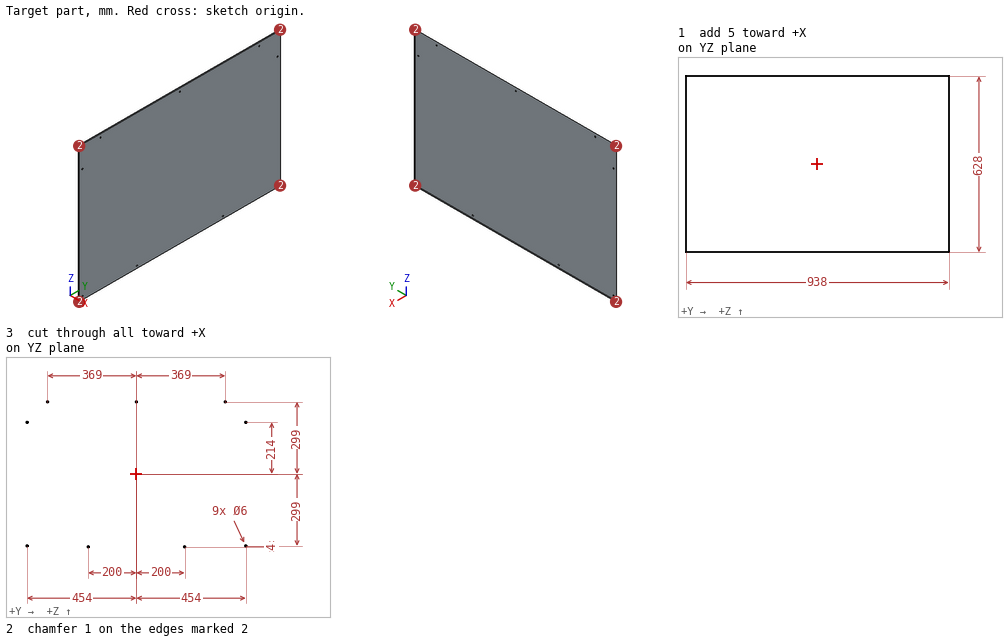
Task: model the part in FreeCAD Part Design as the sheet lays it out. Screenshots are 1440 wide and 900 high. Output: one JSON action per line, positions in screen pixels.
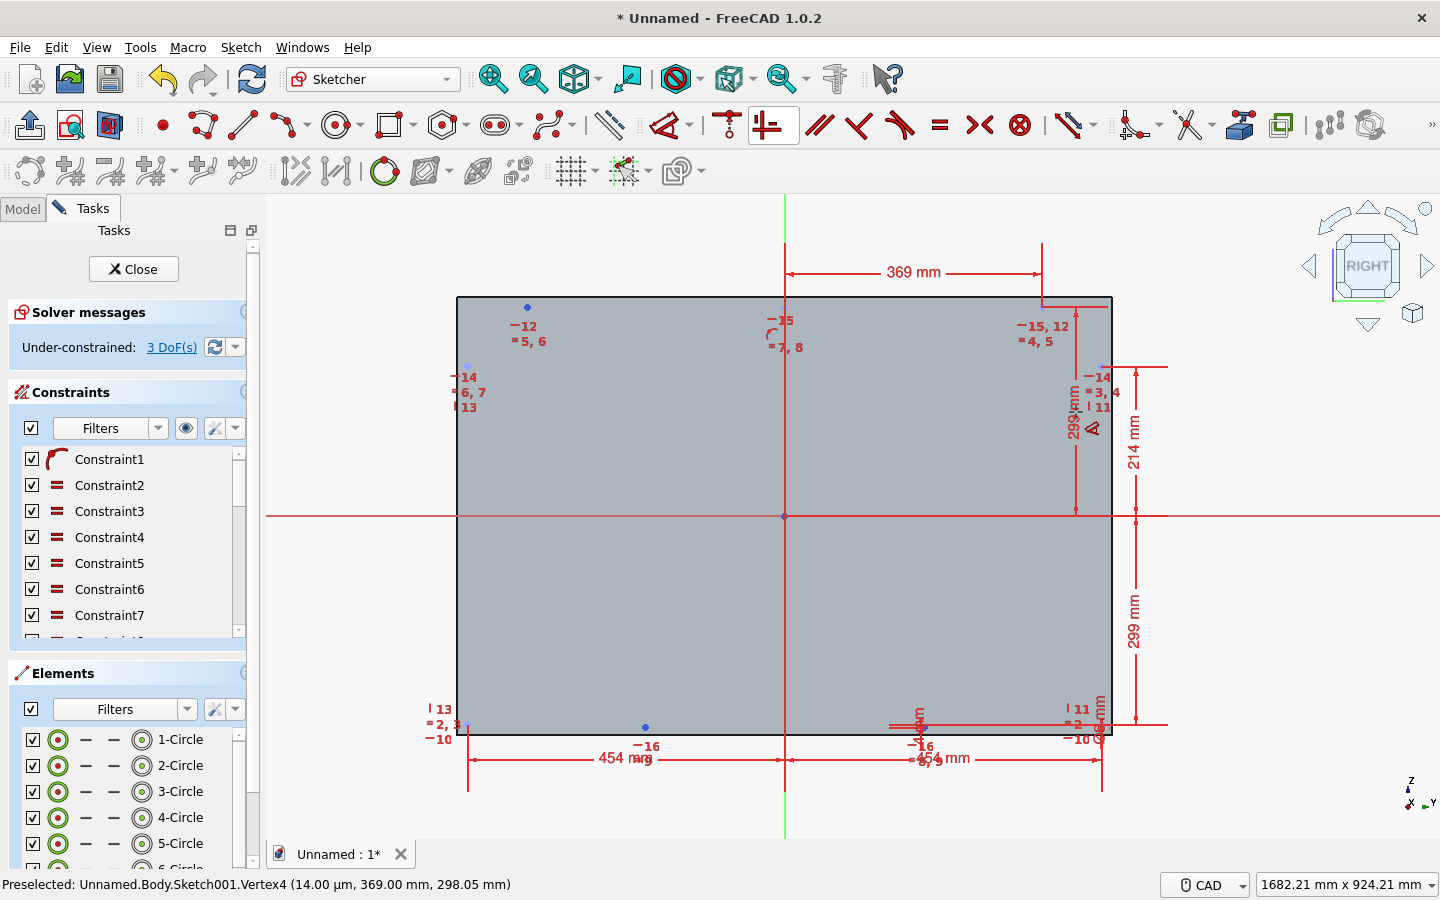
{"action": "left_click", "coordinate": [527, 307]}
{"action": "left_click", "coordinate": [656, 273]}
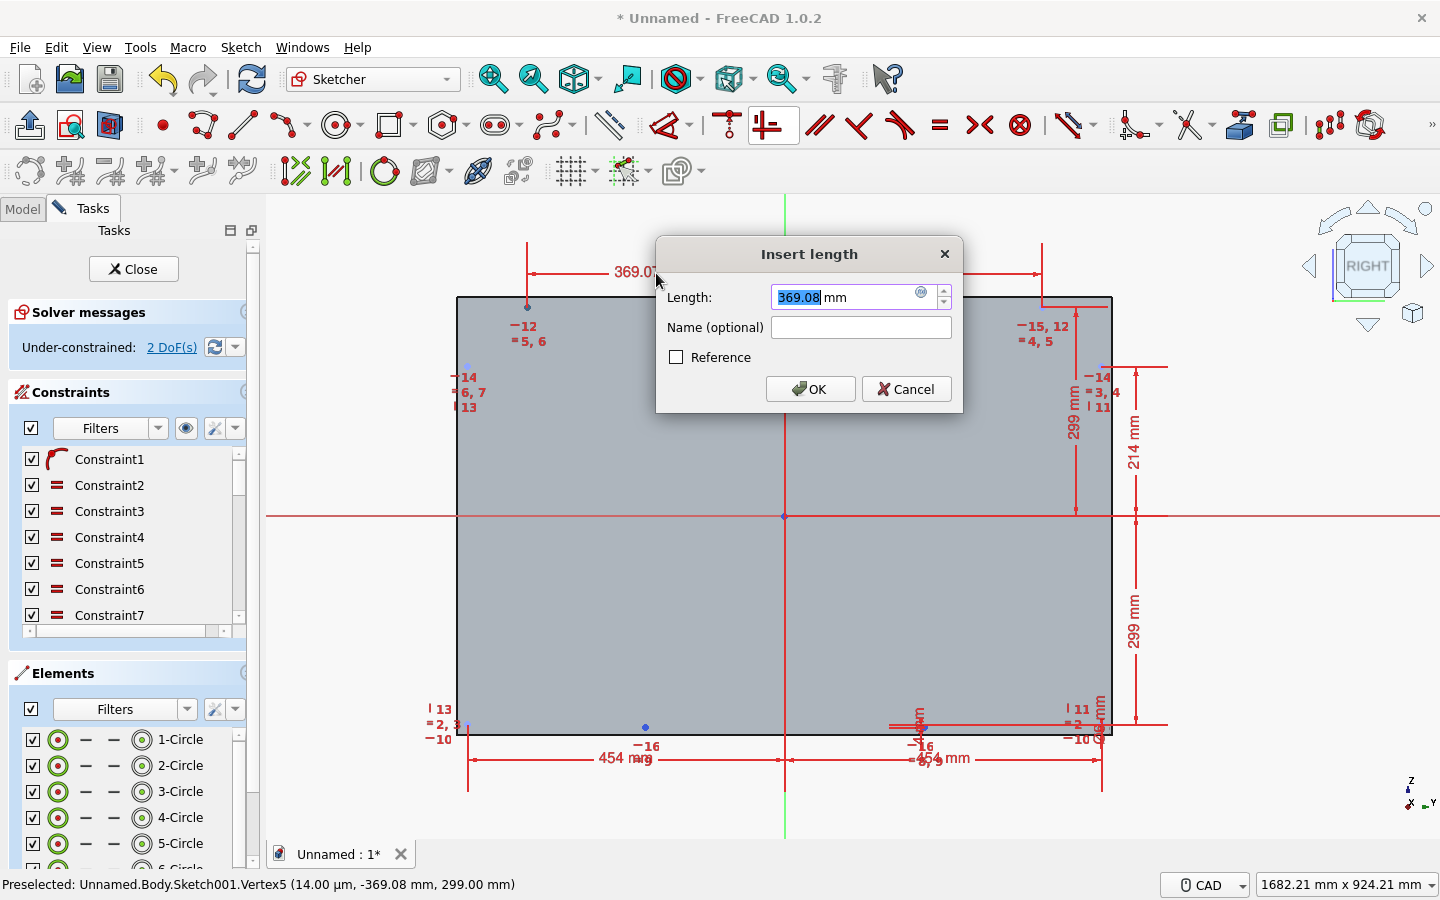
{"action": "type", "text": "369"}
{"action": "key", "text": "Return"}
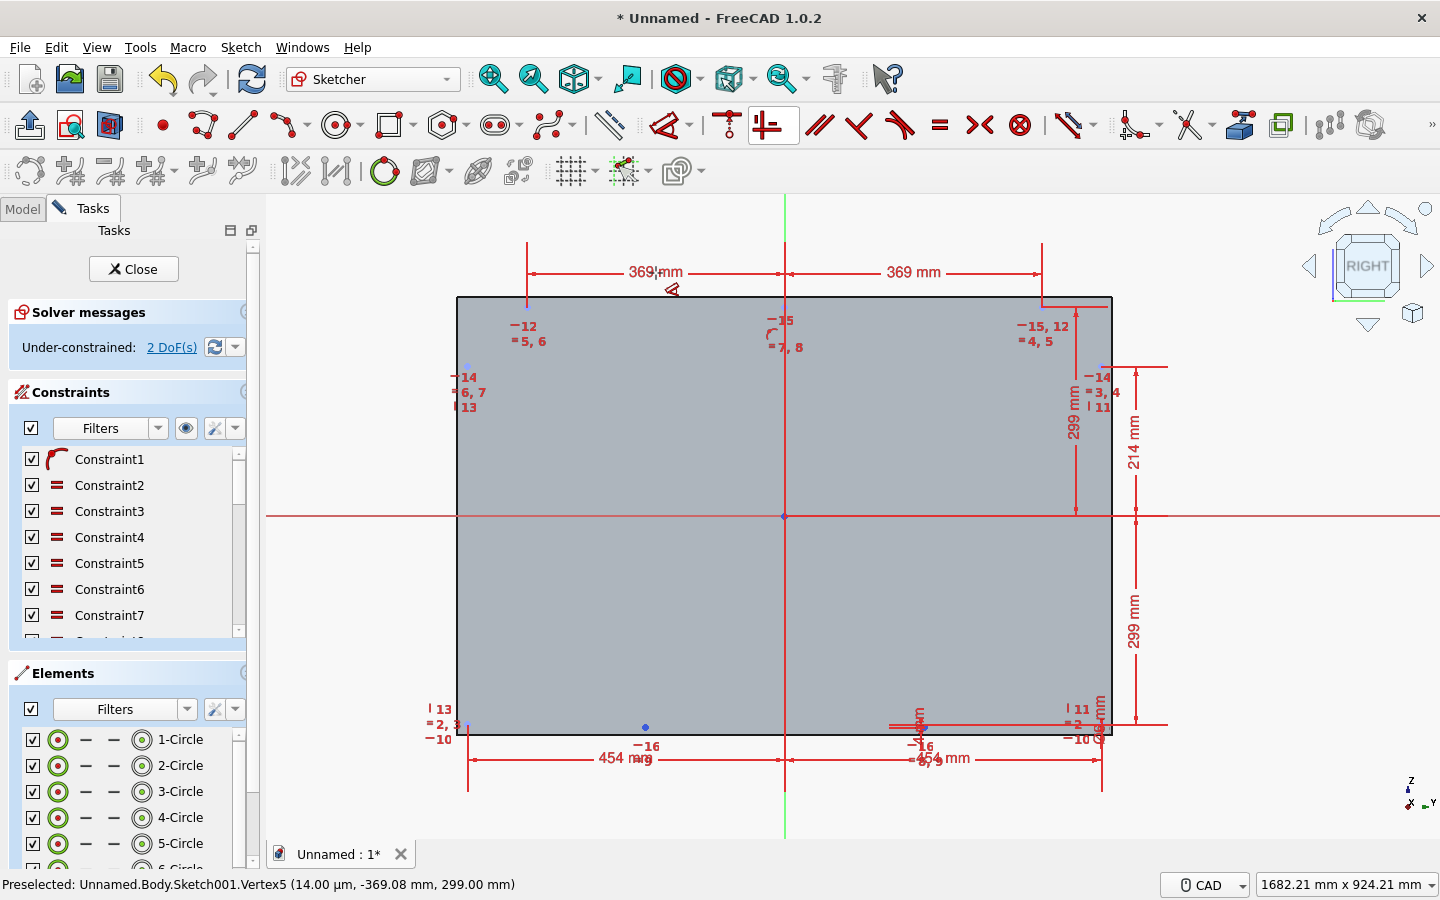
{"action": "left_click", "coordinate": [924, 728]}
{"action": "left_click", "coordinate": [854, 762]}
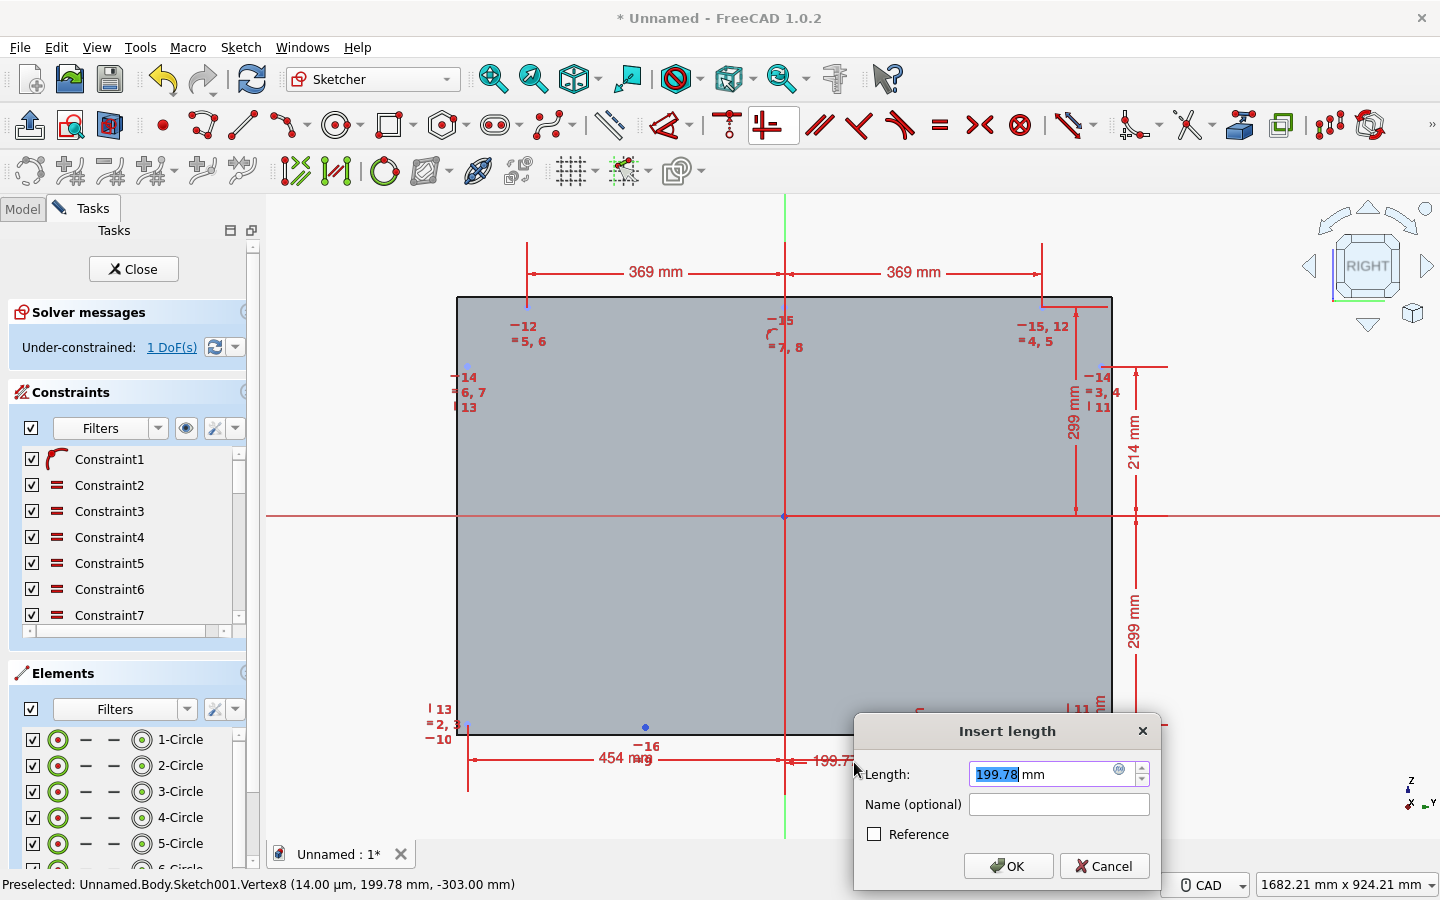
{"action": "type", "text": "200"}
{"action": "key", "text": "Return"}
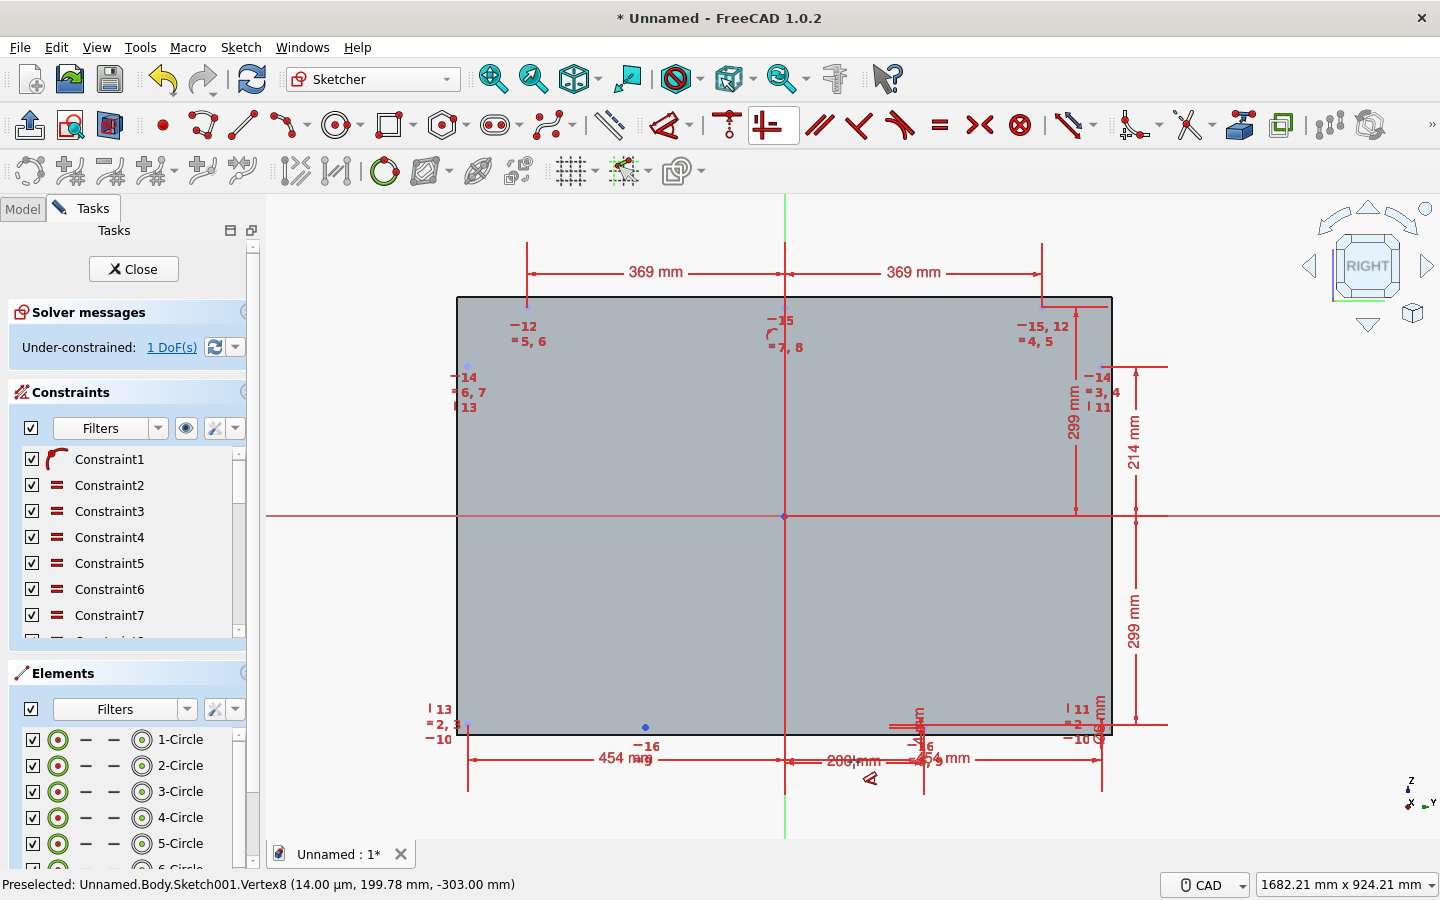
{"action": "left_click", "coordinate": [645, 728]}
{"action": "left_click", "coordinate": [715, 762]}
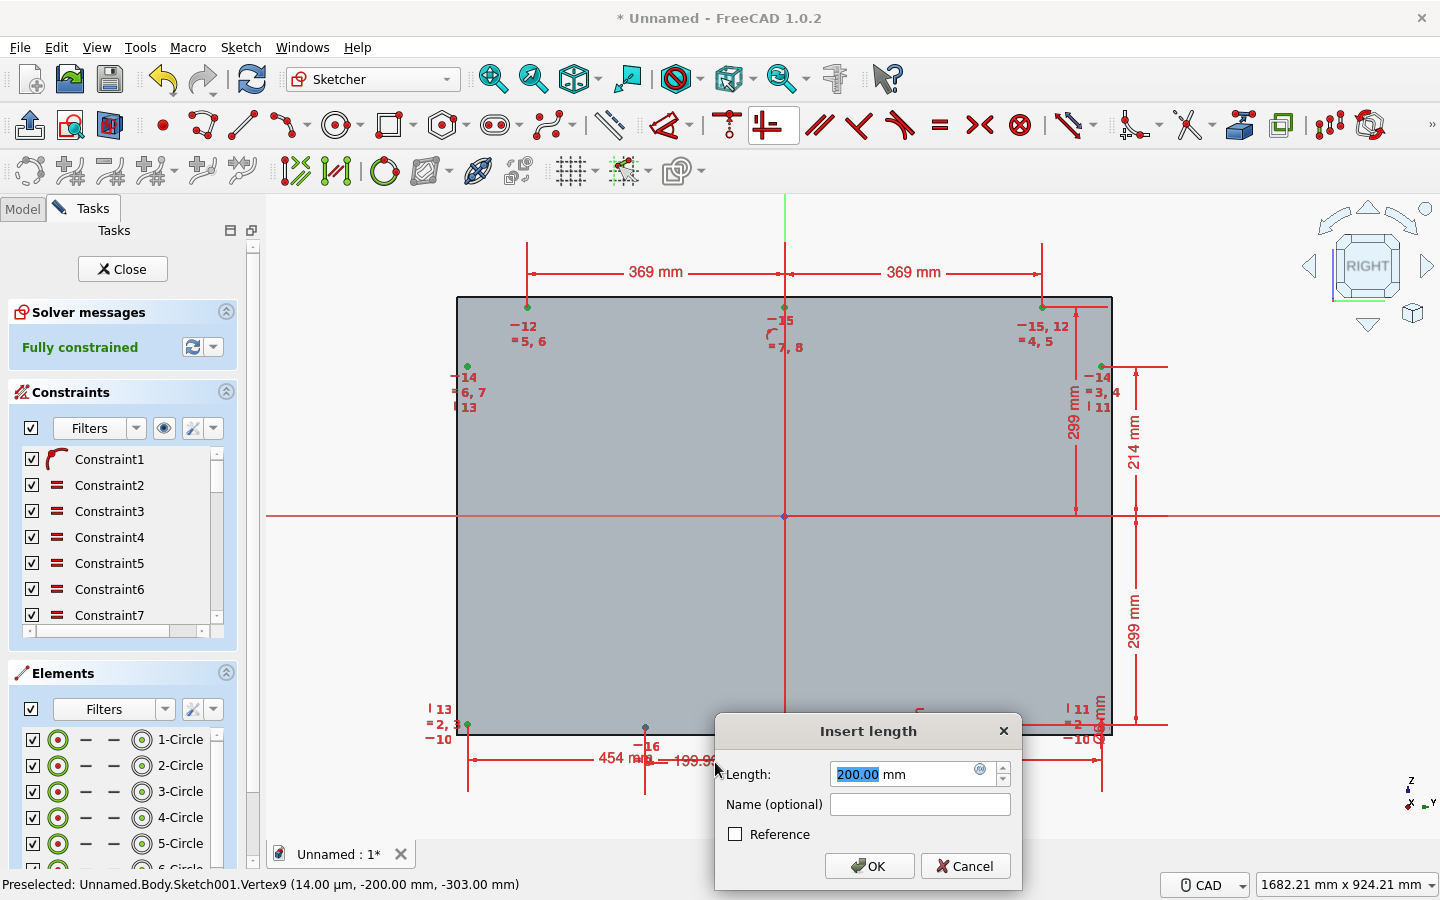
{"action": "type", "text": "200"}
{"action": "key", "text": "Return"}
{"action": "key", "text": "Escape"}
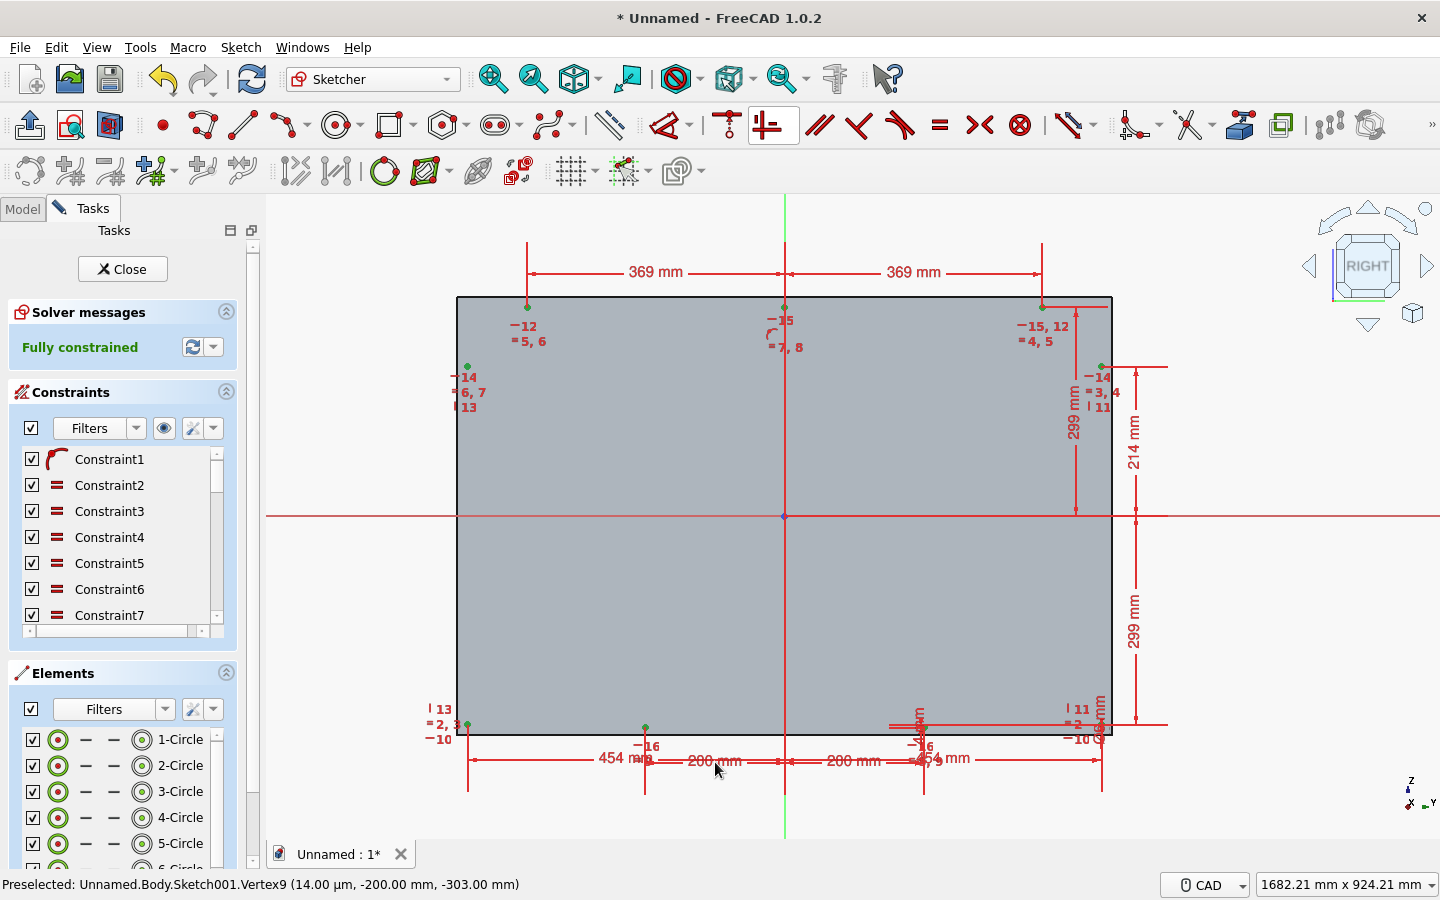
{"action": "left_click", "coordinate": [123, 269]}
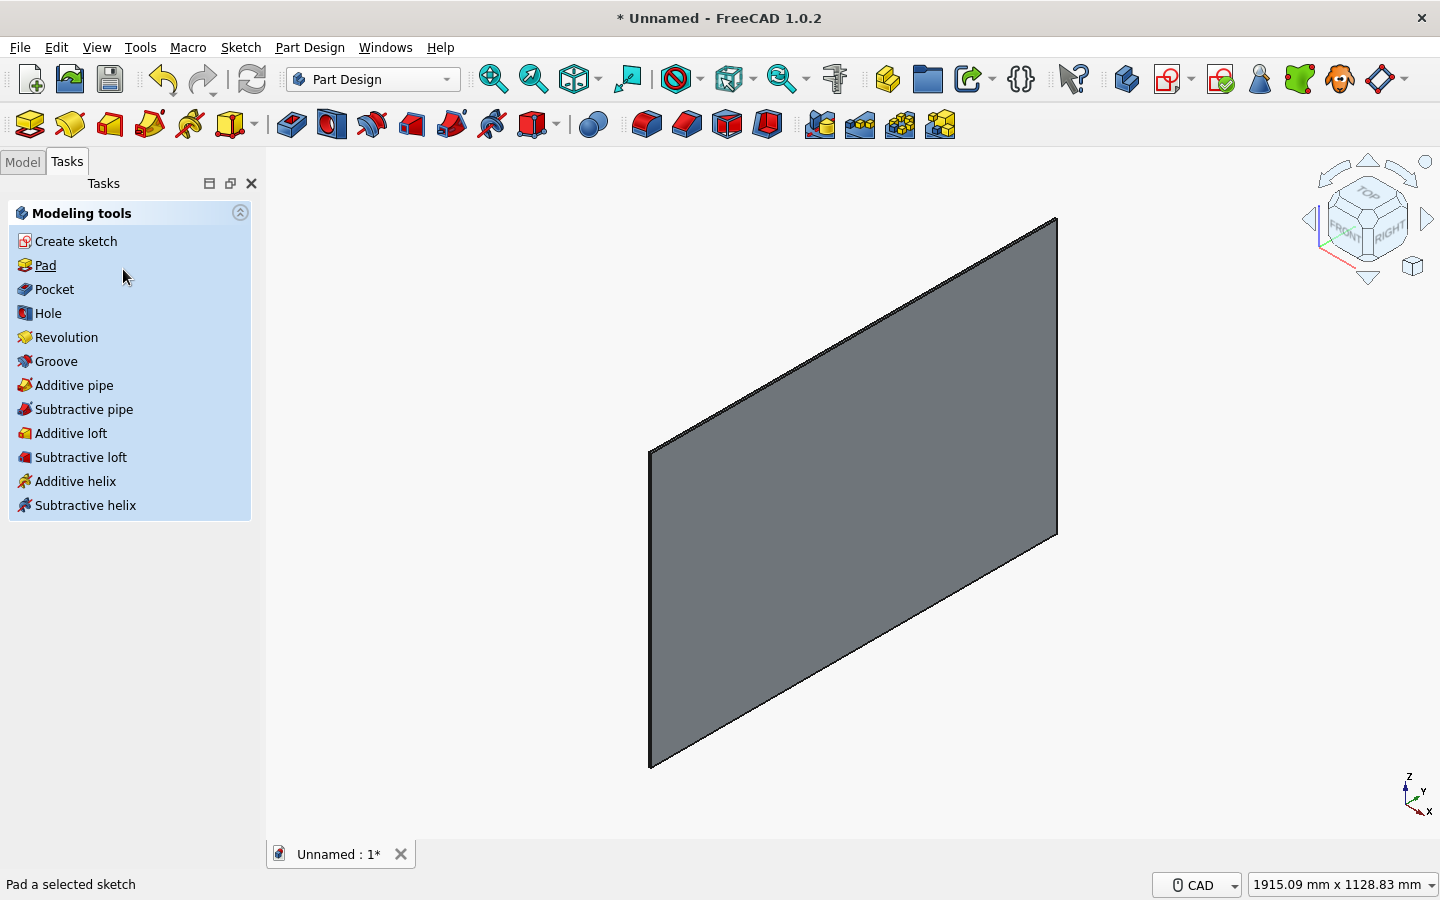
{"action": "left_click", "coordinate": [292, 124]}